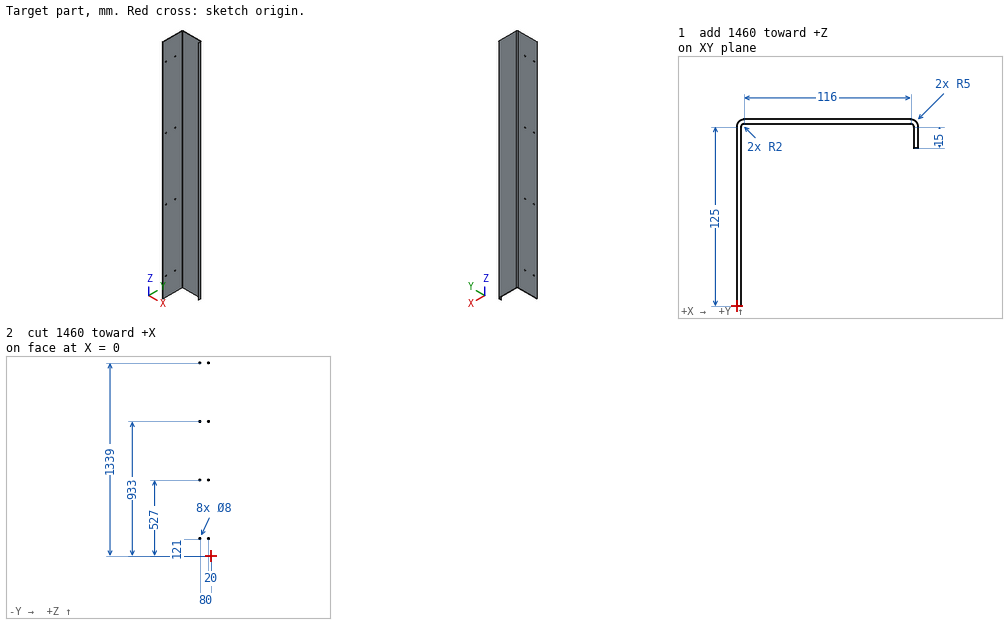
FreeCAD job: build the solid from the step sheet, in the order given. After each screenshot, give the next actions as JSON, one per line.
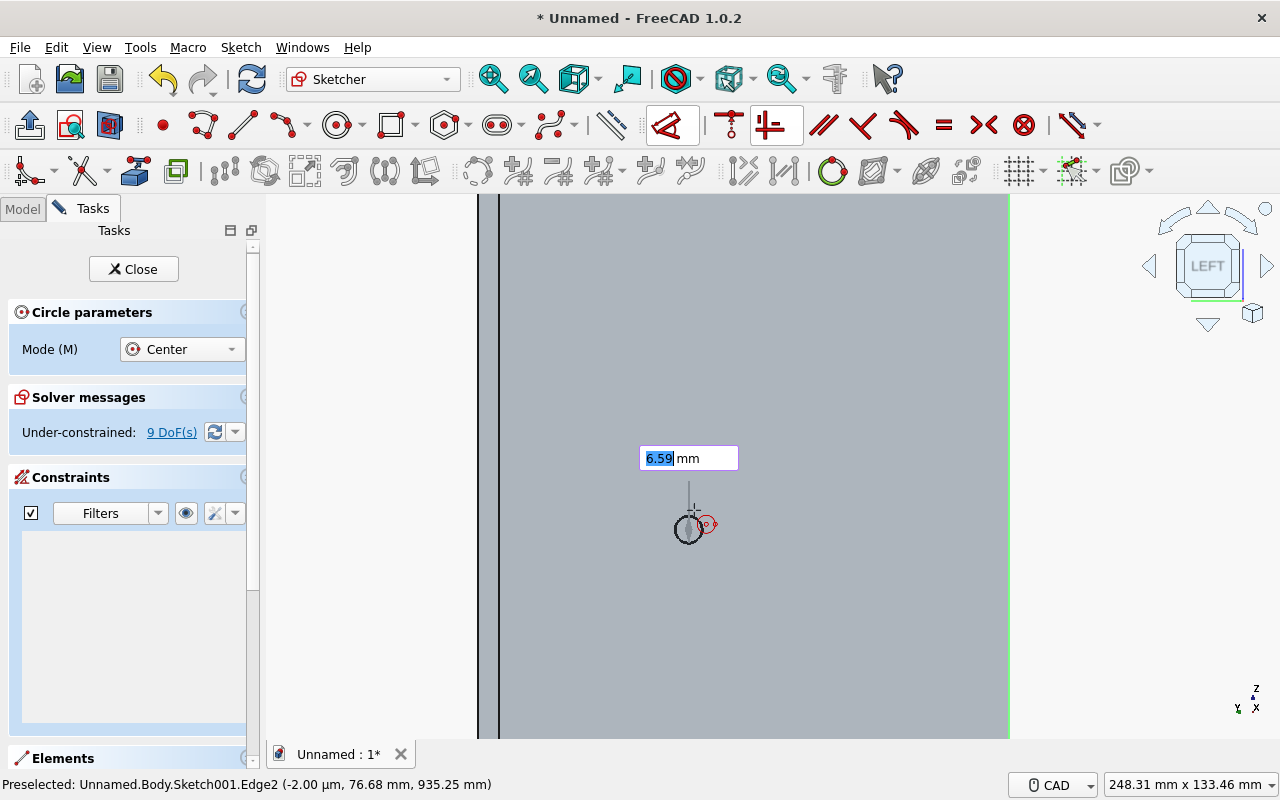
{"action": "left_click", "coordinate": [694, 506]}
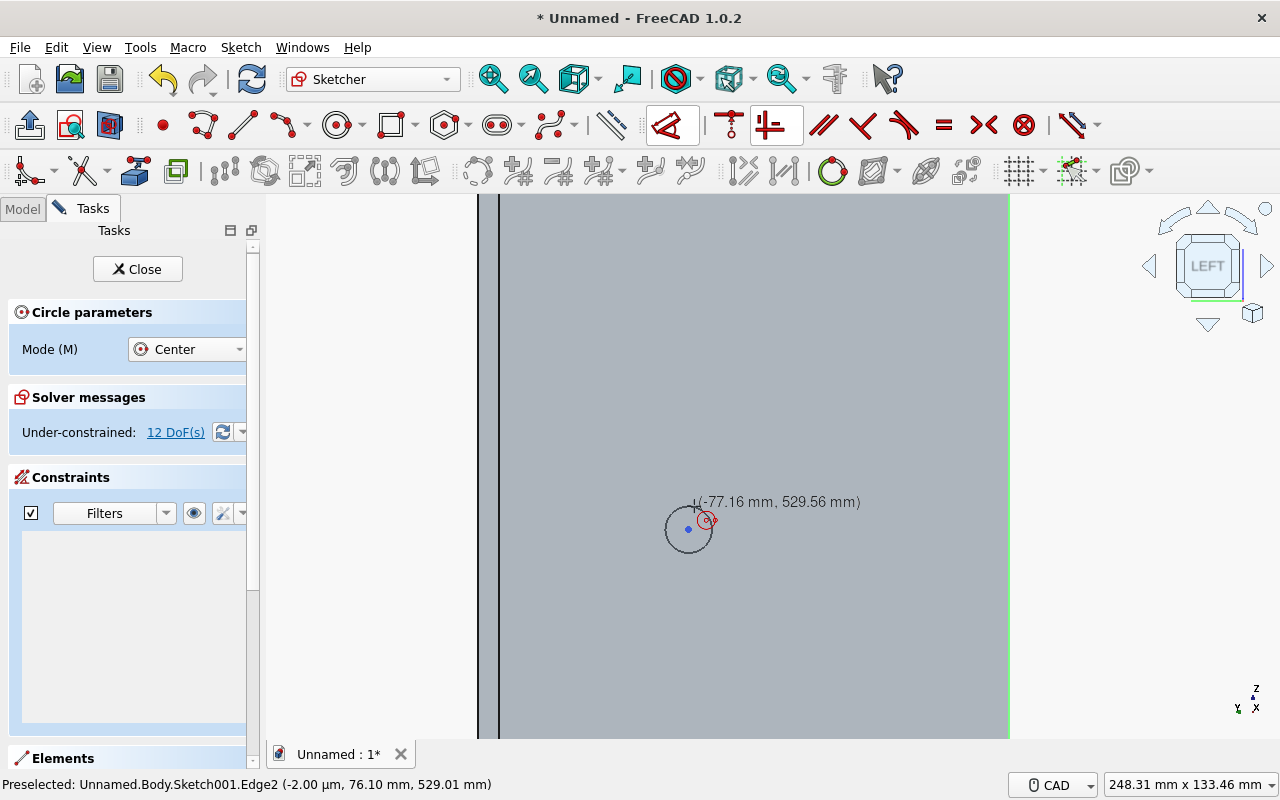
{"action": "scroll", "coordinate": [696, 501], "scroll_direction": "down", "scroll_amount": 14}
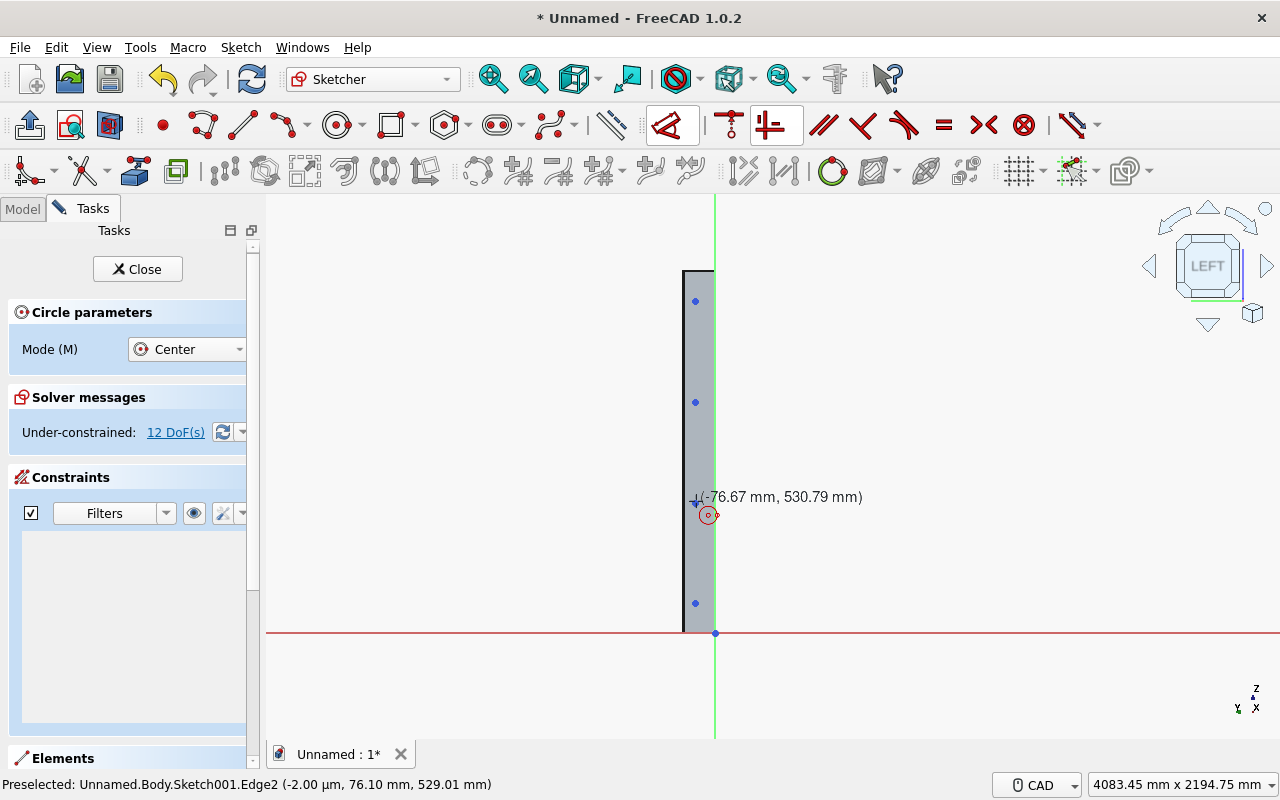
{"action": "scroll", "coordinate": [710, 603], "scroll_direction": "up", "scroll_amount": 16}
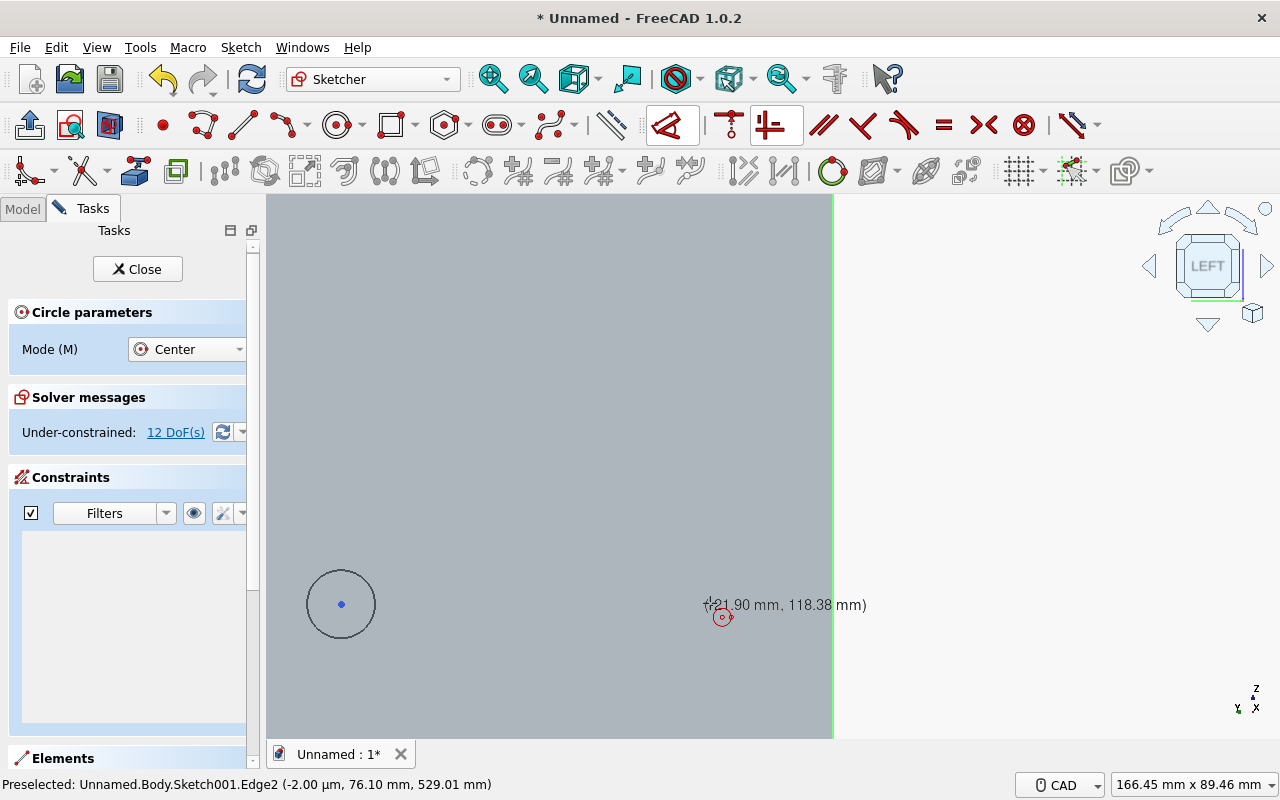
{"action": "scroll", "coordinate": [711, 636], "scroll_direction": "down", "scroll_amount": 15}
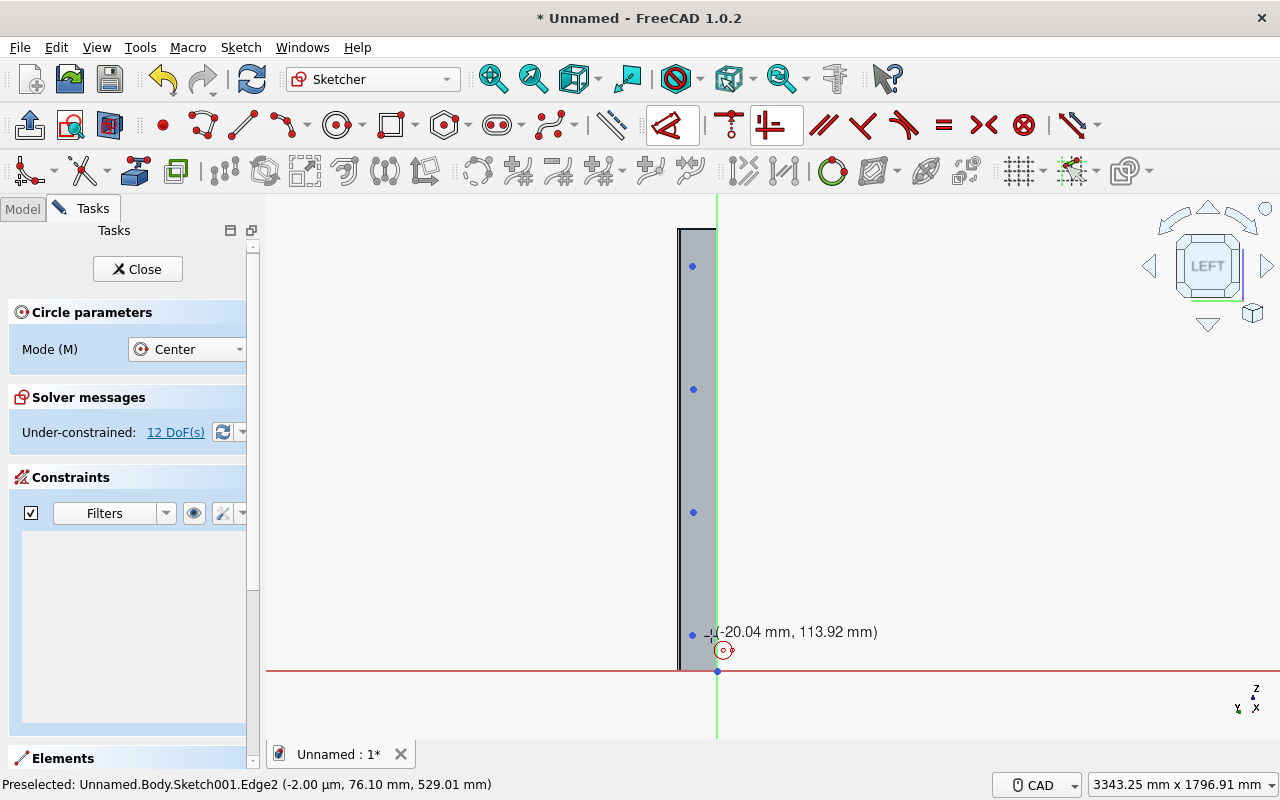
{"action": "scroll", "coordinate": [711, 635], "scroll_direction": "up", "scroll_amount": 5}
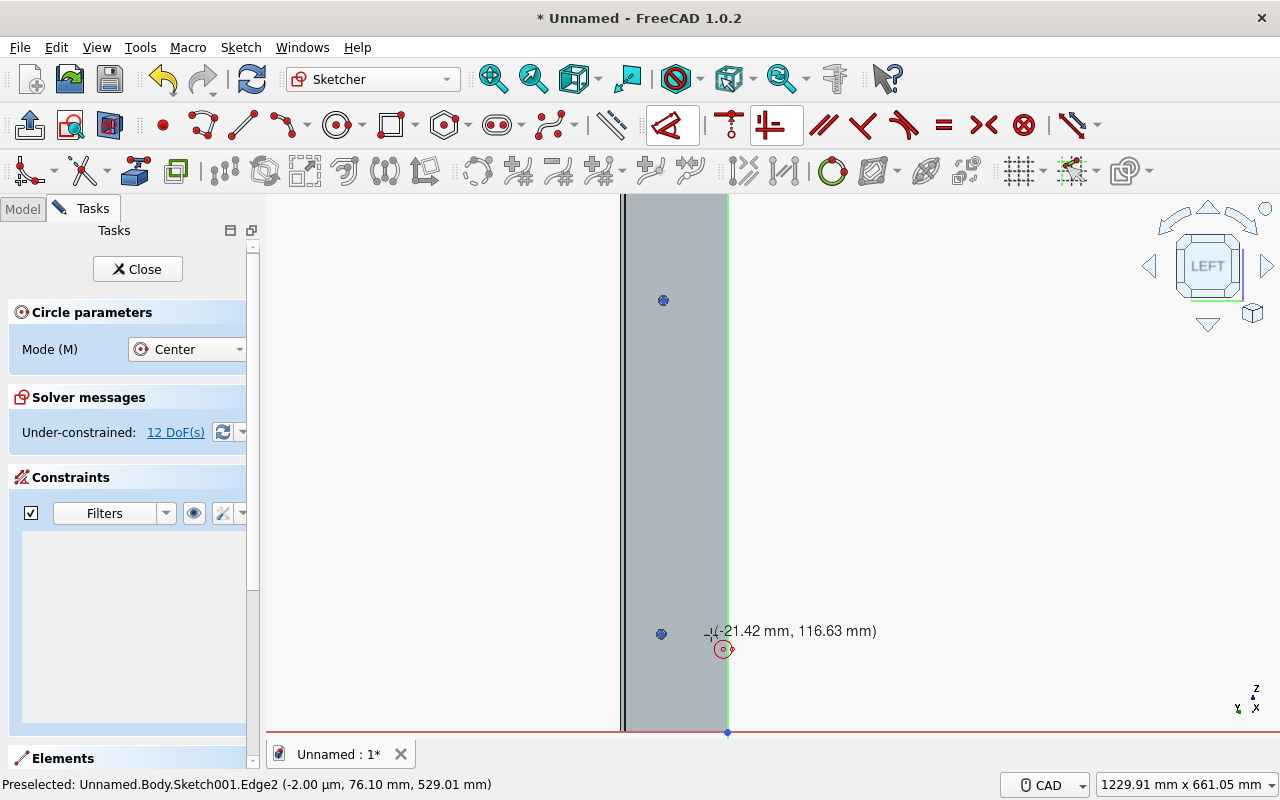
{"action": "left_click", "coordinate": [711, 633]}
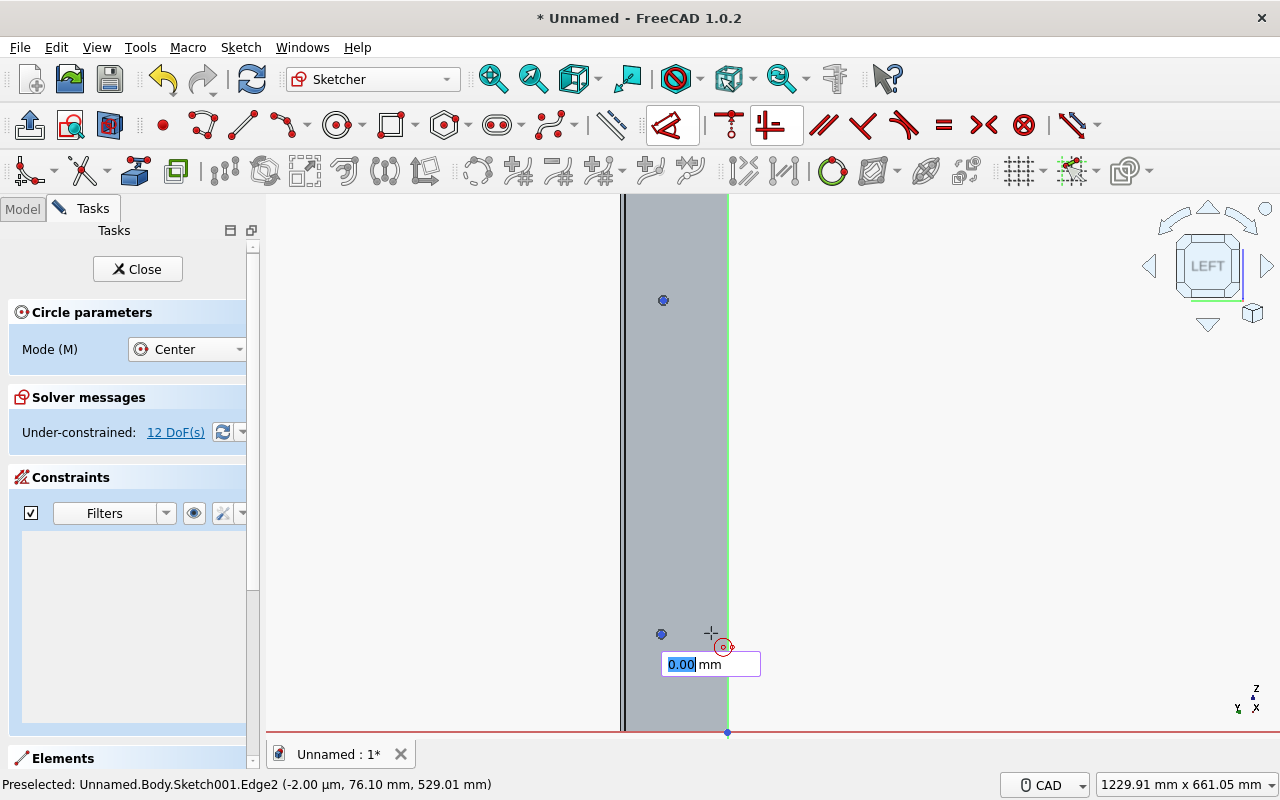
{"action": "scroll", "coordinate": [714, 630], "scroll_direction": "up", "scroll_amount": 8}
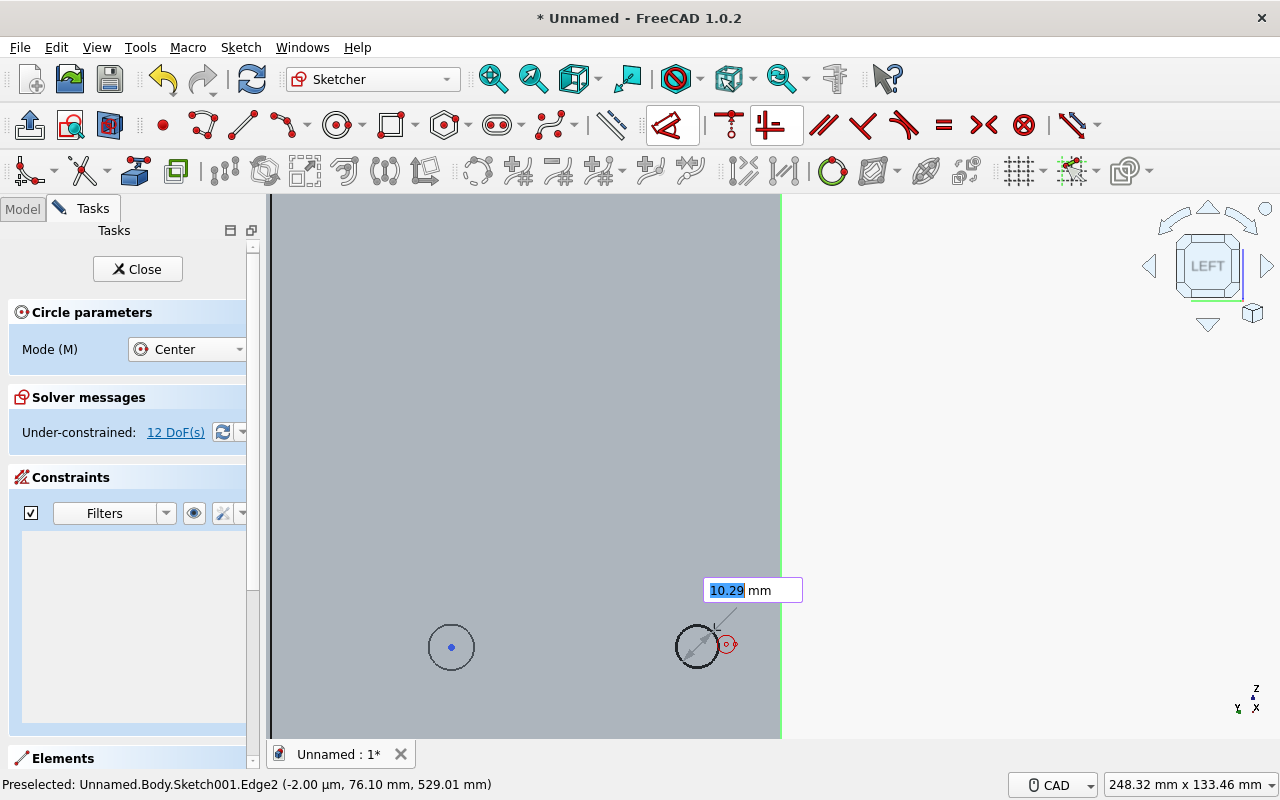
{"action": "left_click", "coordinate": [711, 629]}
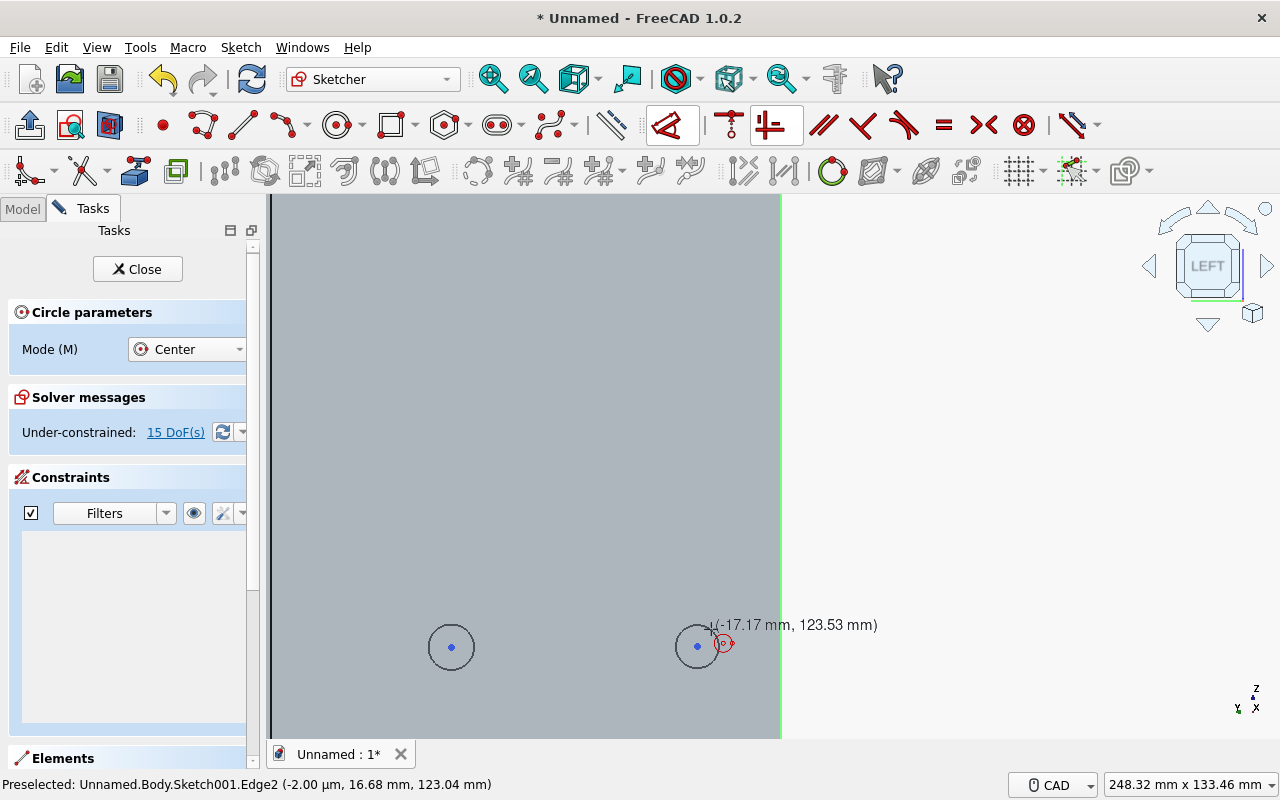
{"action": "scroll", "coordinate": [711, 601], "scroll_direction": "down", "scroll_amount": 14}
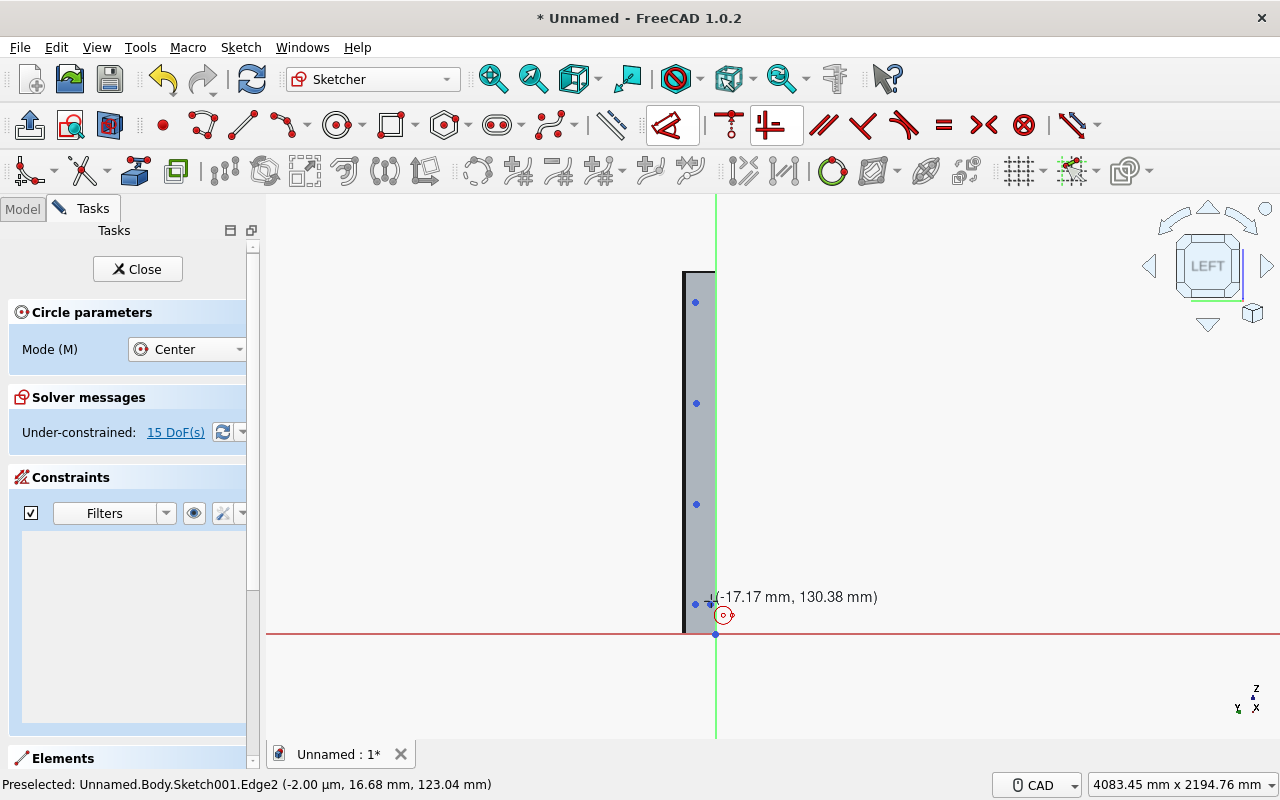
{"action": "scroll", "coordinate": [711, 302], "scroll_direction": "up", "scroll_amount": 16}